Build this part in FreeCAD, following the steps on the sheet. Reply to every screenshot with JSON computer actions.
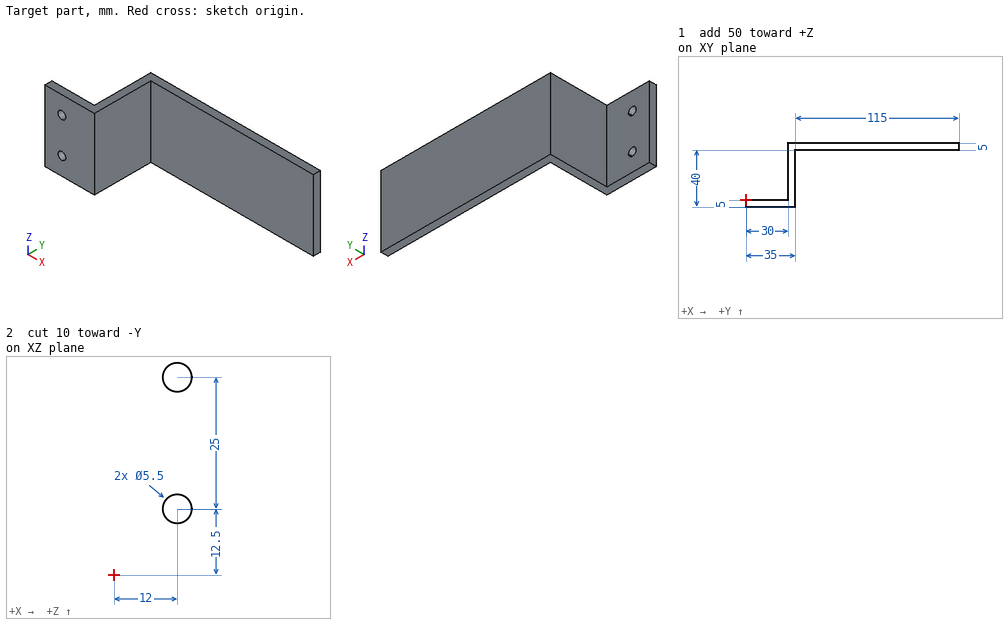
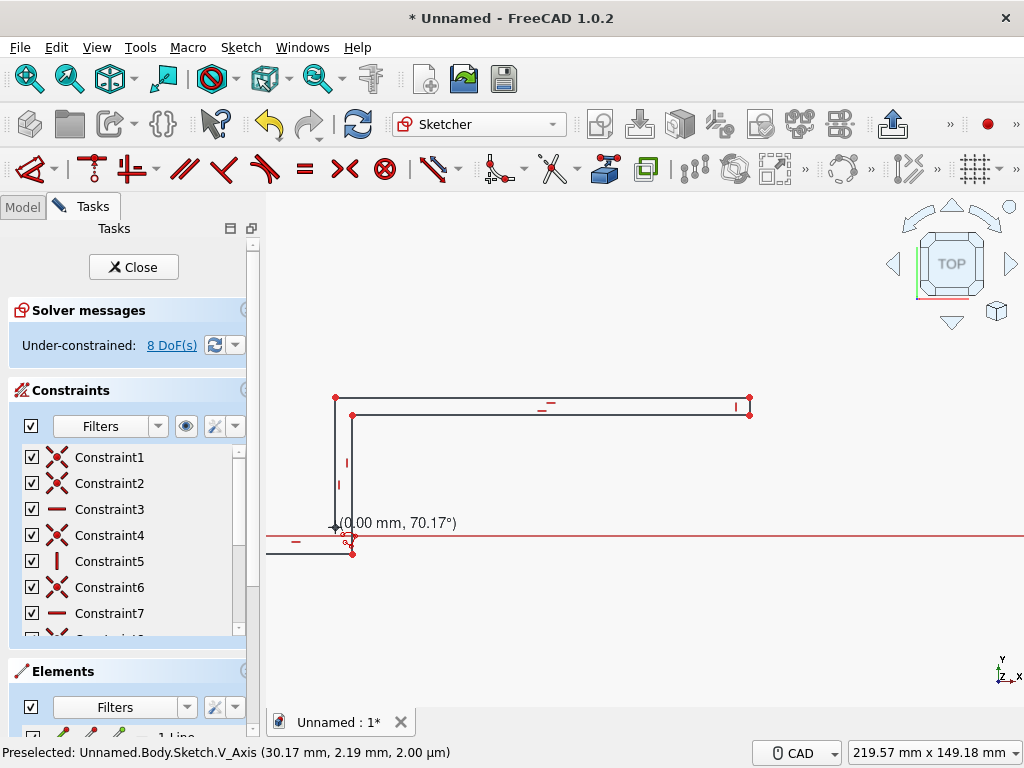
{"action": "scroll", "coordinate": [859, 334], "scroll_direction": "down", "scroll_amount": 1}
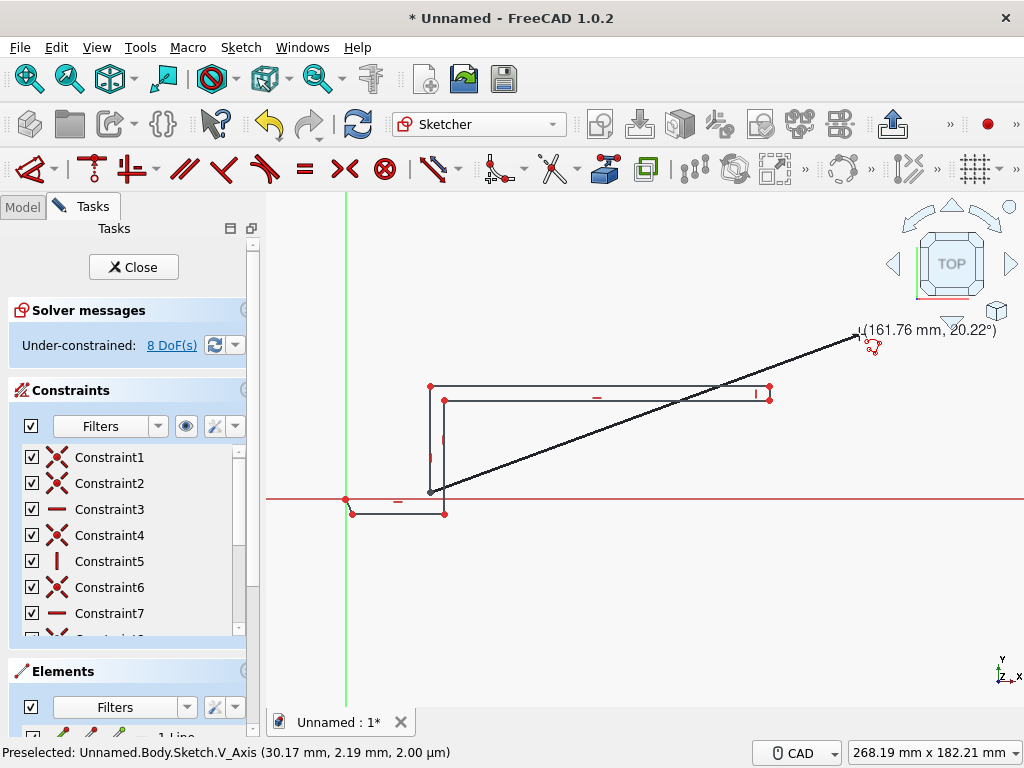
{"action": "scroll", "coordinate": [346, 499], "scroll_direction": "up", "scroll_amount": 5}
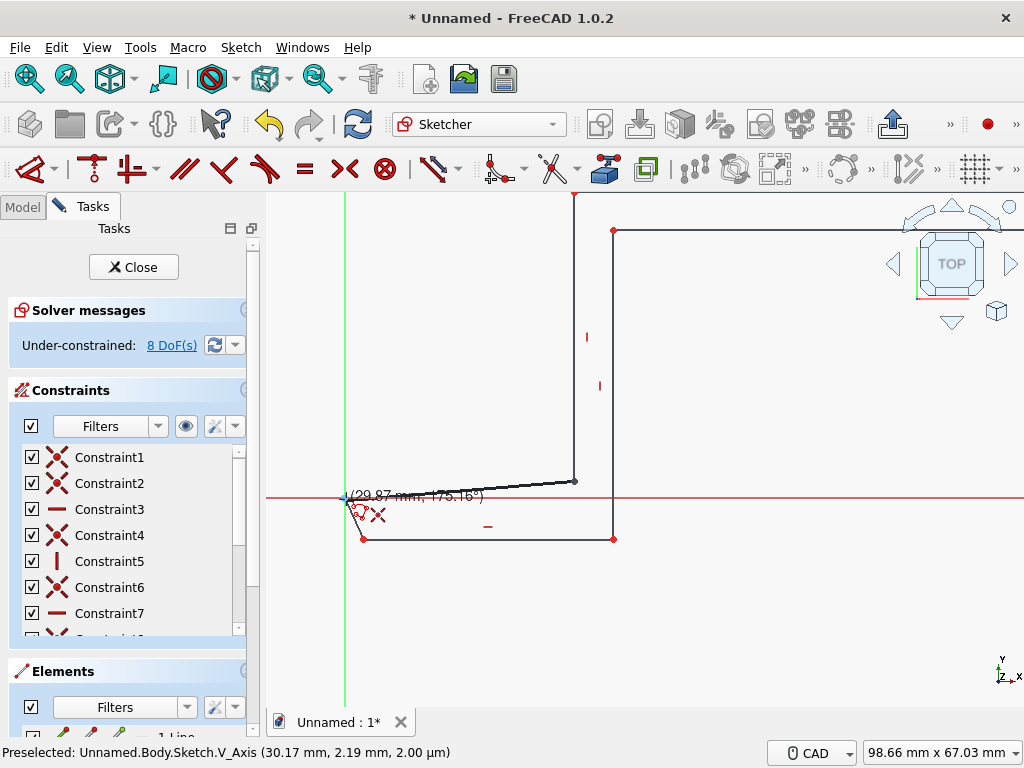
{"action": "left_click", "coordinate": [345, 498]}
{"action": "key", "text": "Escape"}
{"action": "key", "text": "Escape"}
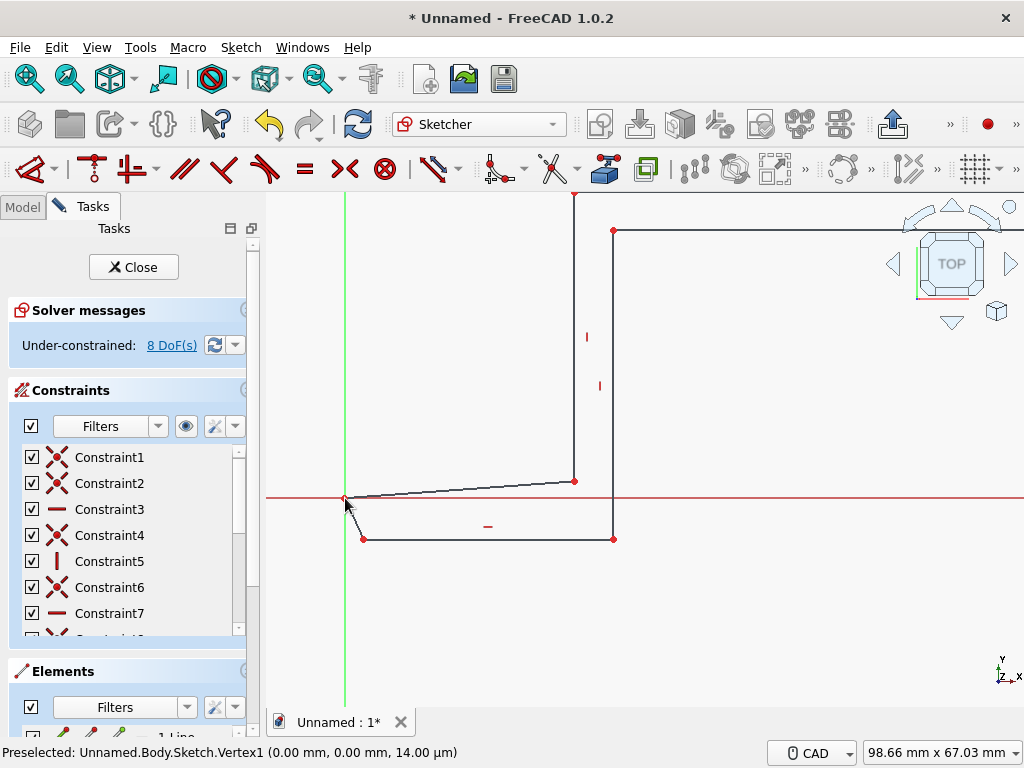
{"action": "left_click", "coordinate": [358, 527]}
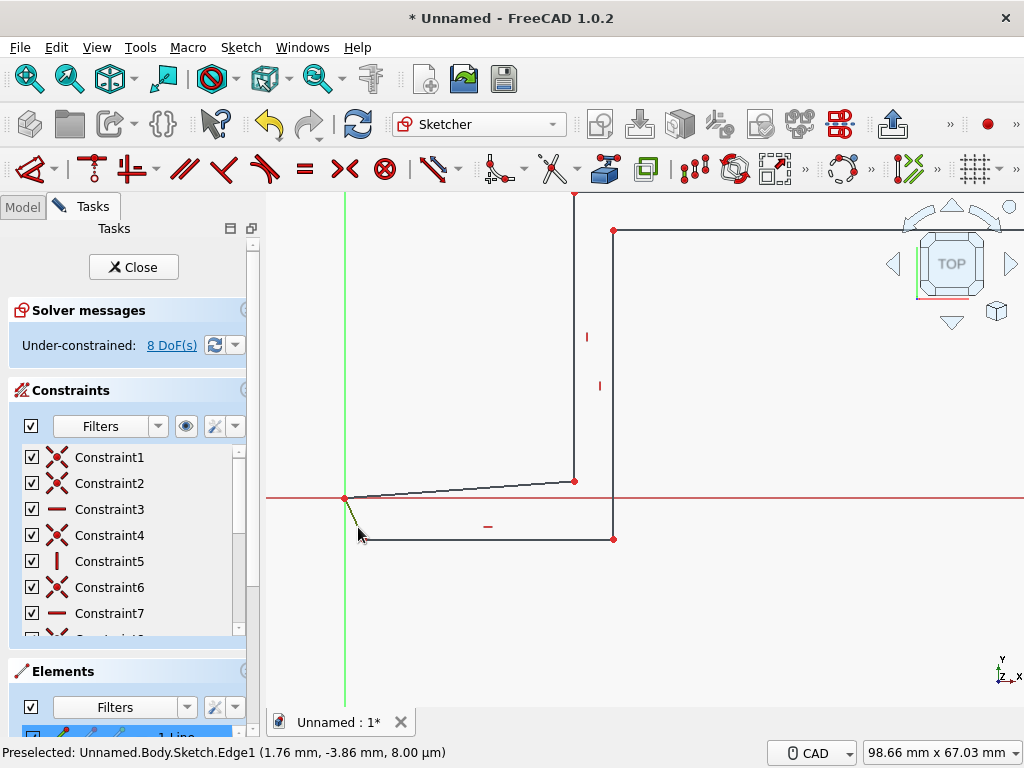
{"action": "left_click", "coordinate": [158, 170]}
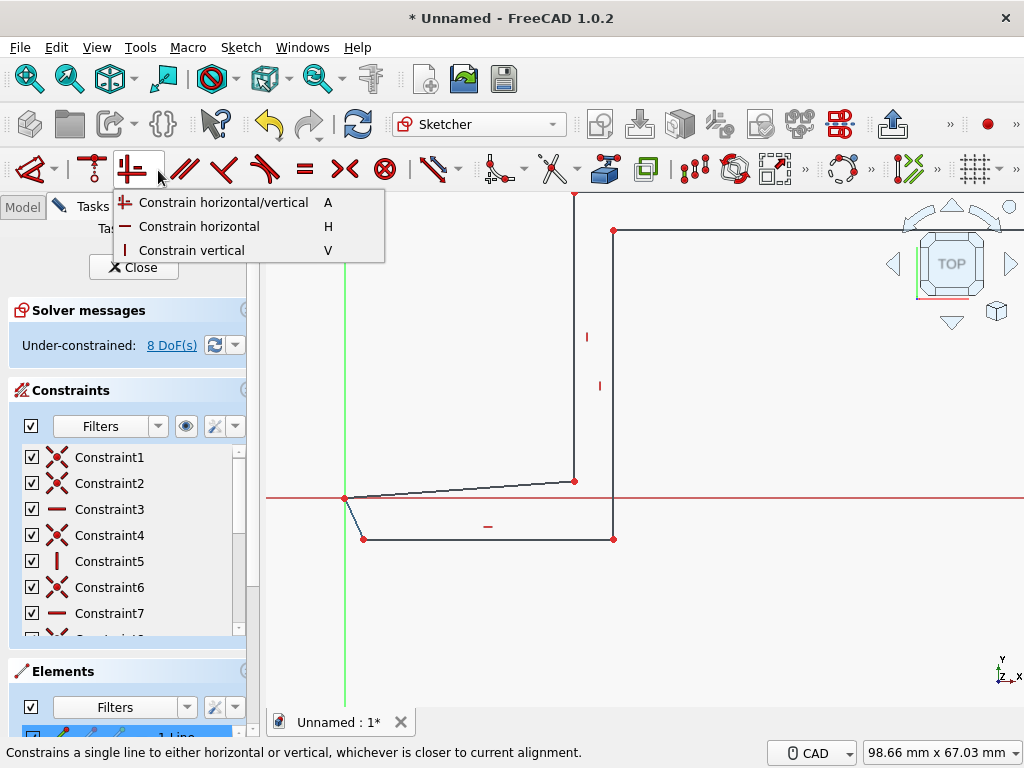
{"action": "left_click", "coordinate": [249, 250]}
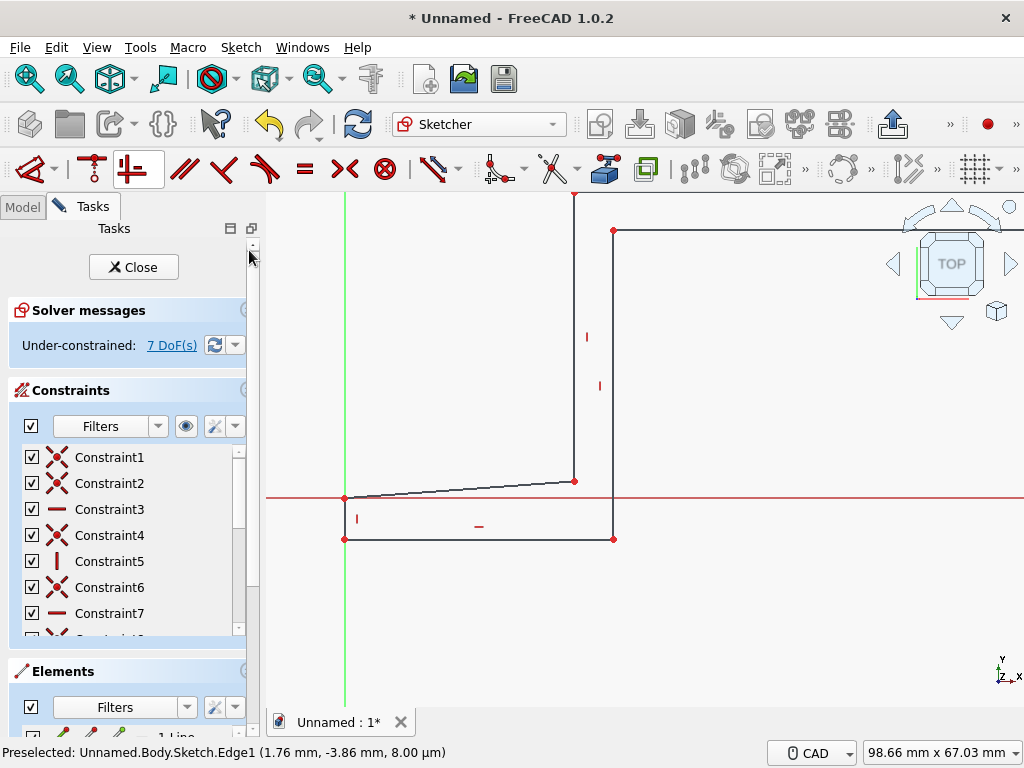
{"action": "left_click", "coordinate": [506, 486]}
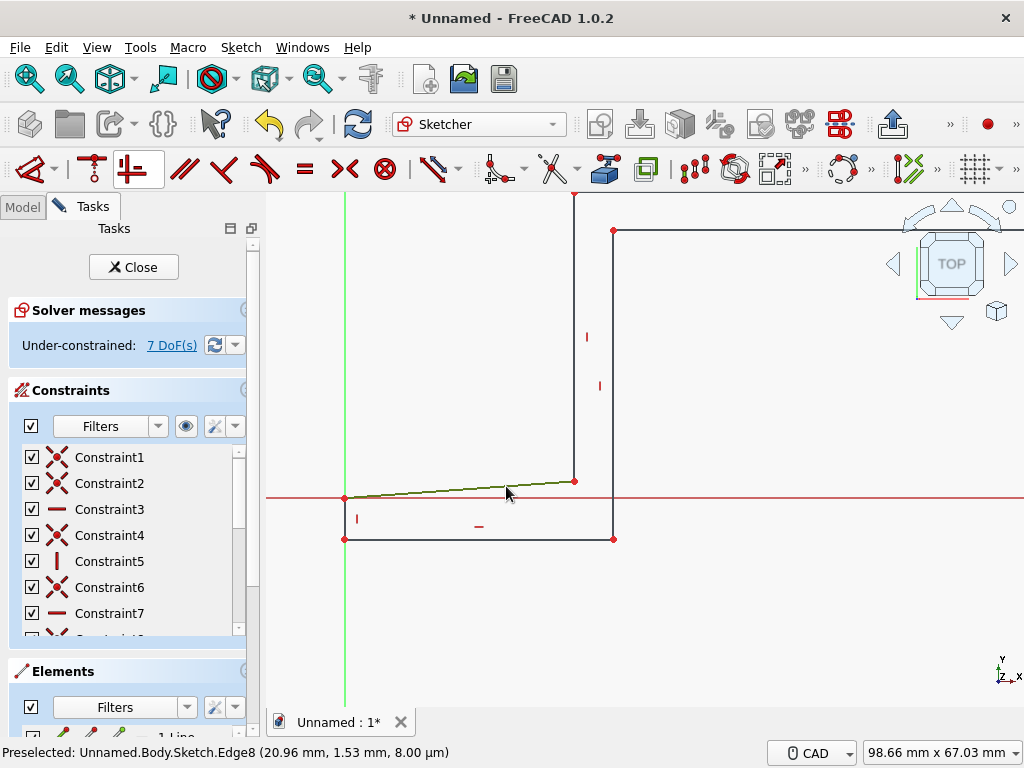
{"action": "left_click", "coordinate": [158, 170]}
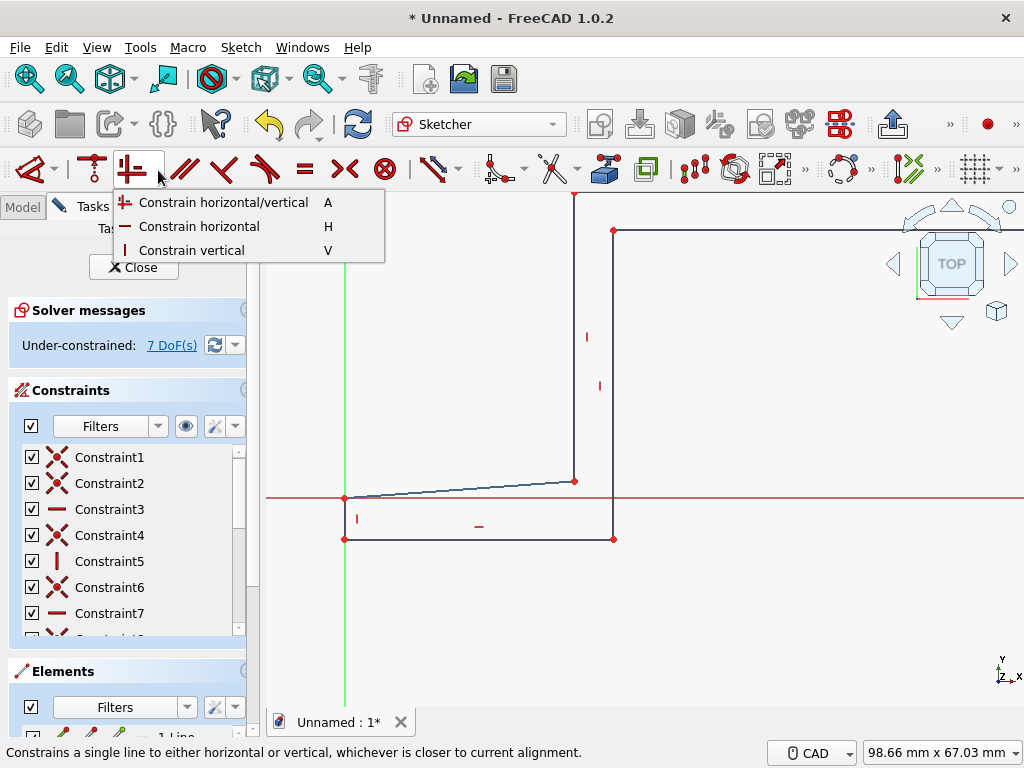
{"action": "left_click", "coordinate": [249, 226]}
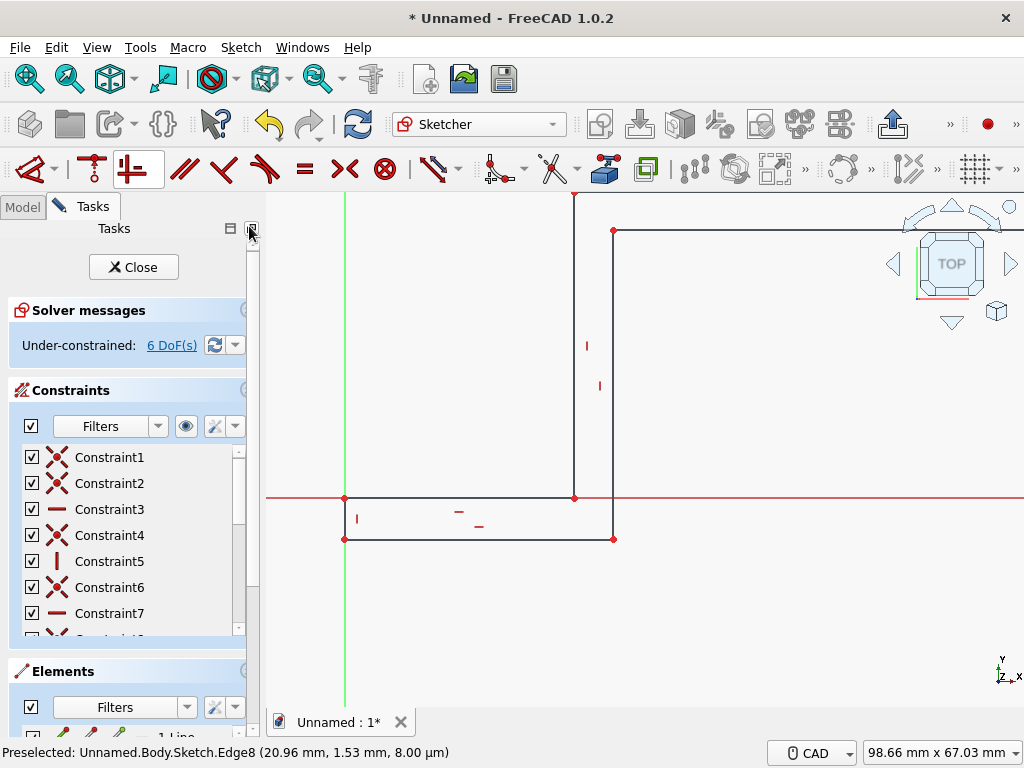
{"action": "left_click", "coordinate": [345, 511]}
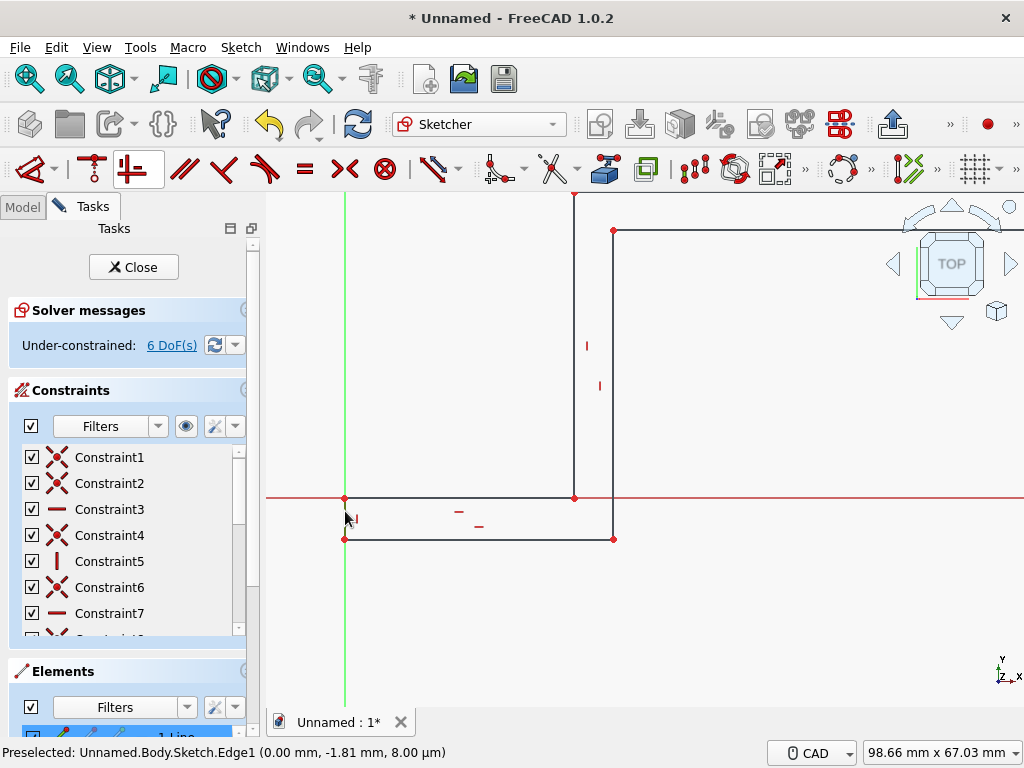
{"action": "key", "text": "i"}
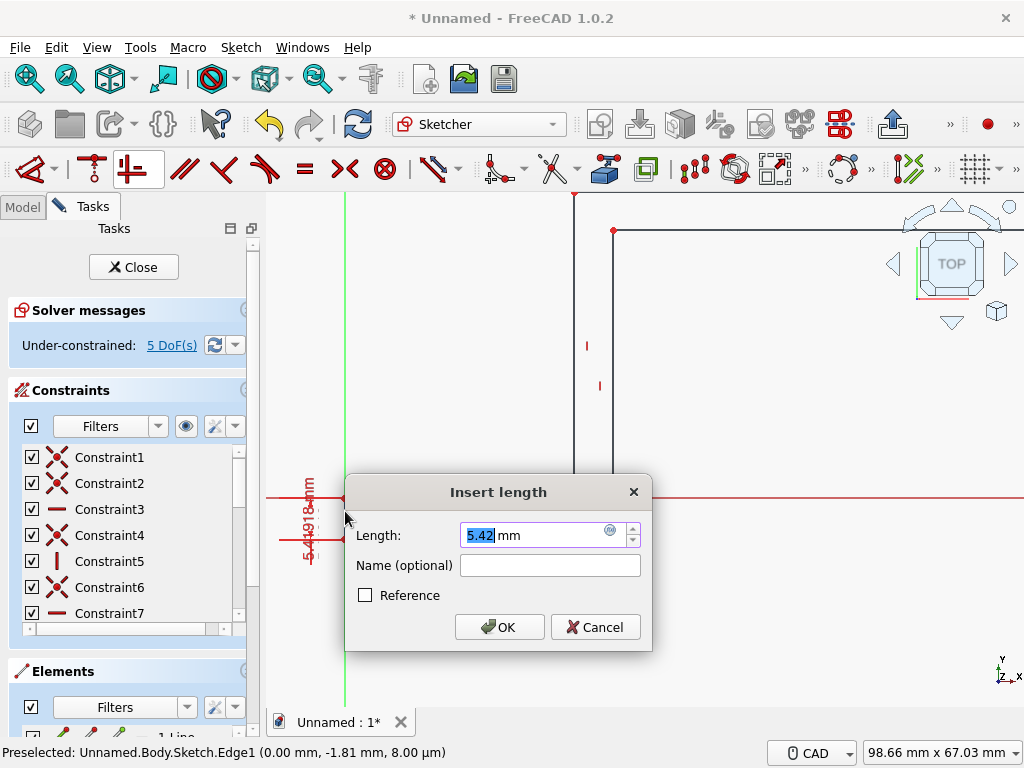
{"action": "type", "text": "5"}
{"action": "key", "text": "Return"}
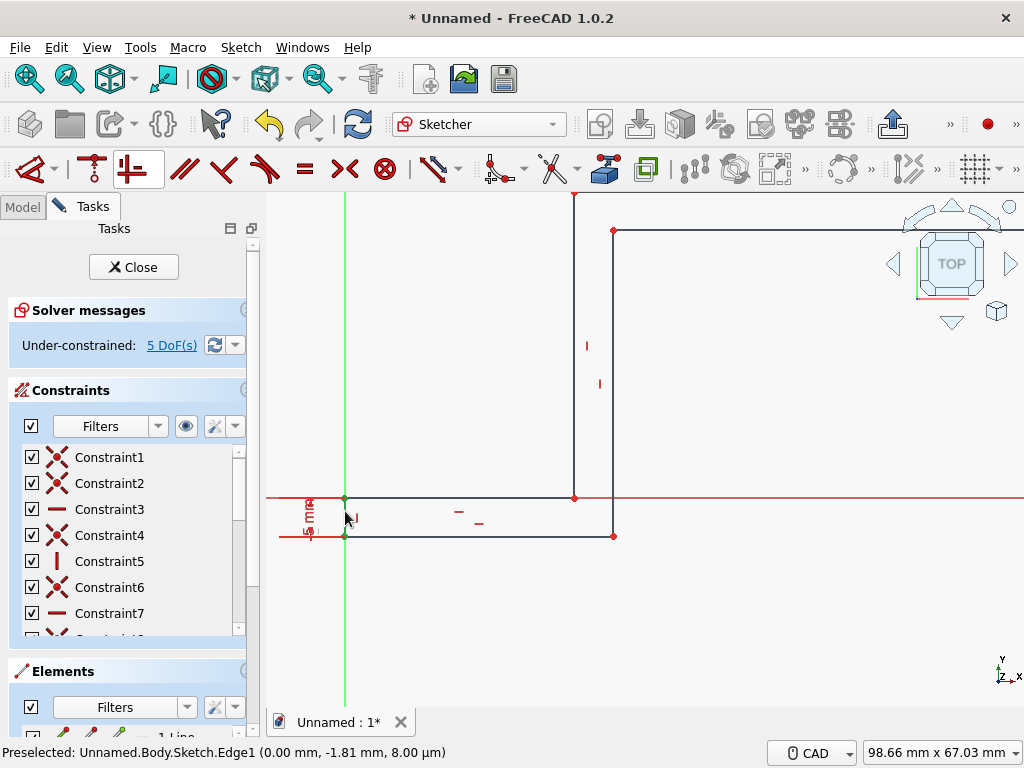
{"action": "scroll", "coordinate": [376, 499], "scroll_direction": "down", "scroll_amount": 5}